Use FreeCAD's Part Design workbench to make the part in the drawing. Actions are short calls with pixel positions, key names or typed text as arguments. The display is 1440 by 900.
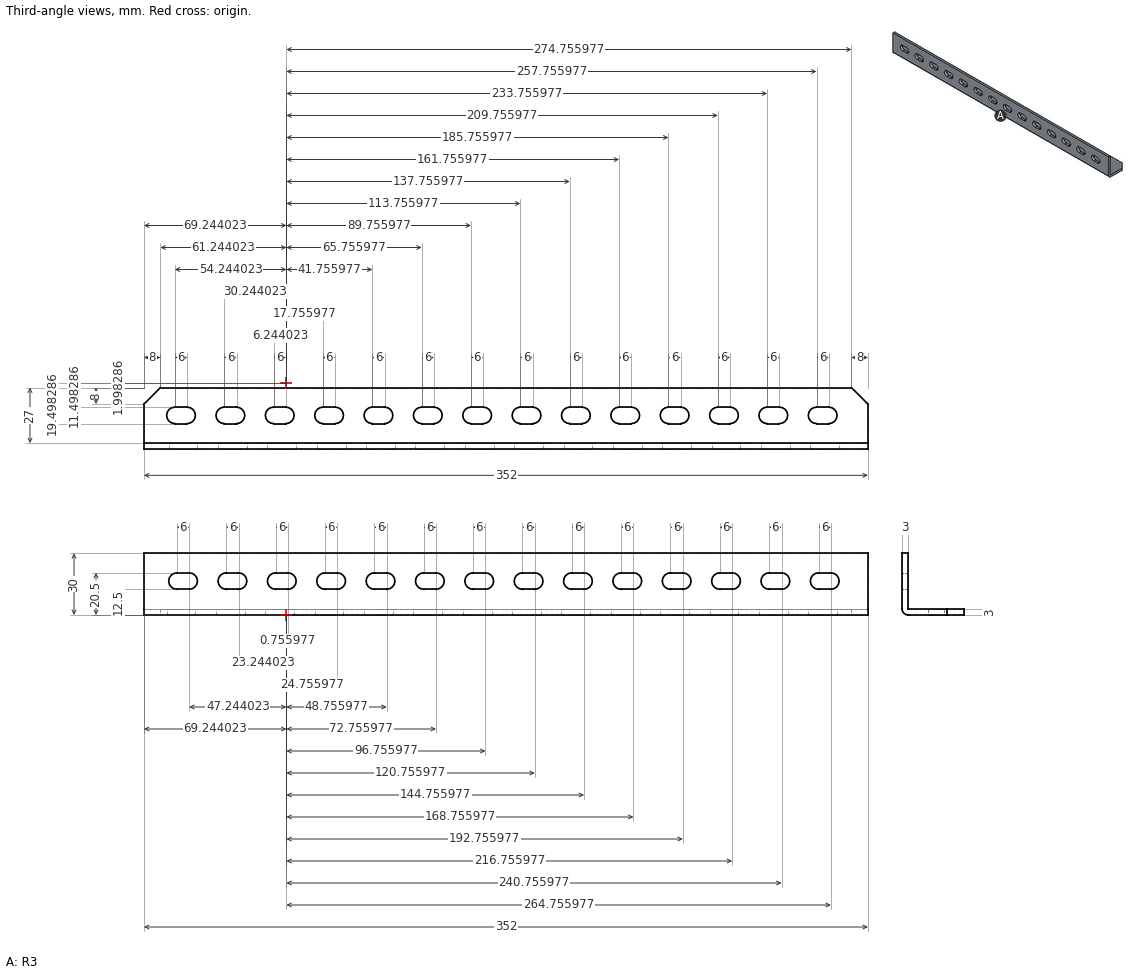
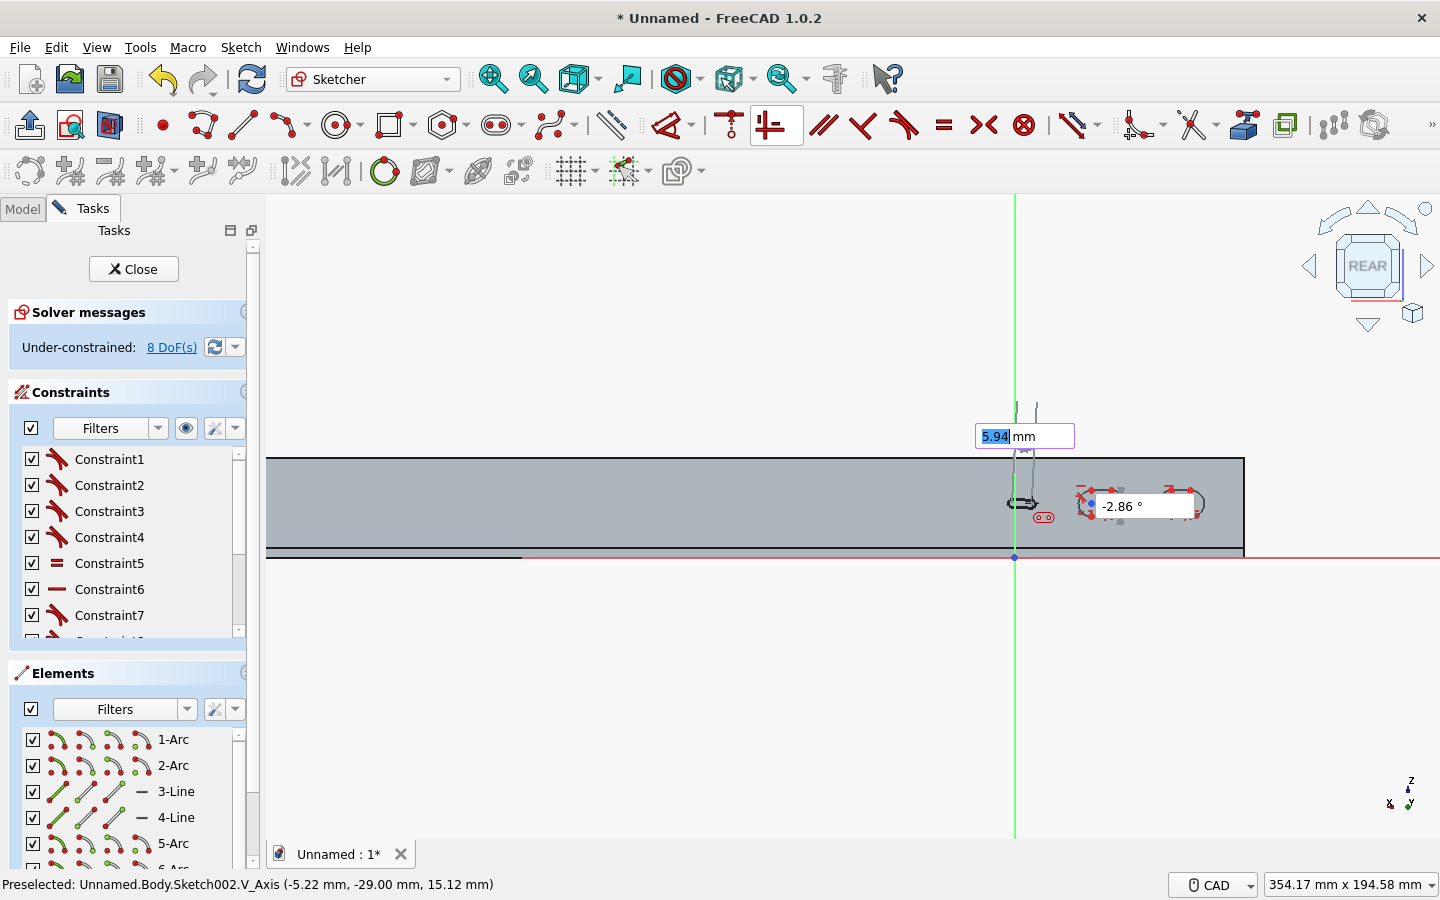
click(1032, 503)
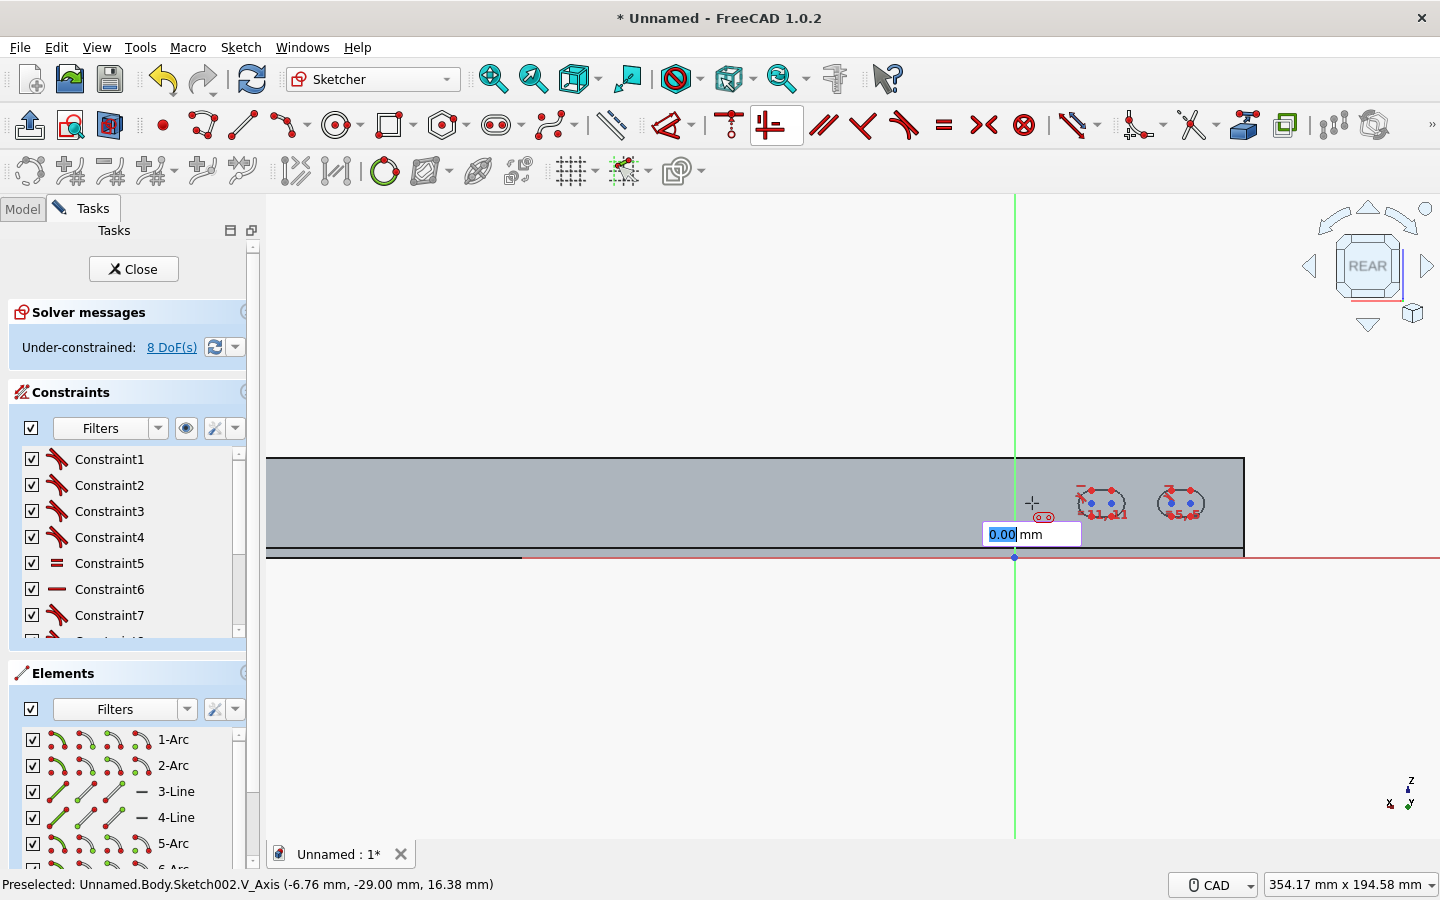
scroll(1025, 516, up, 3)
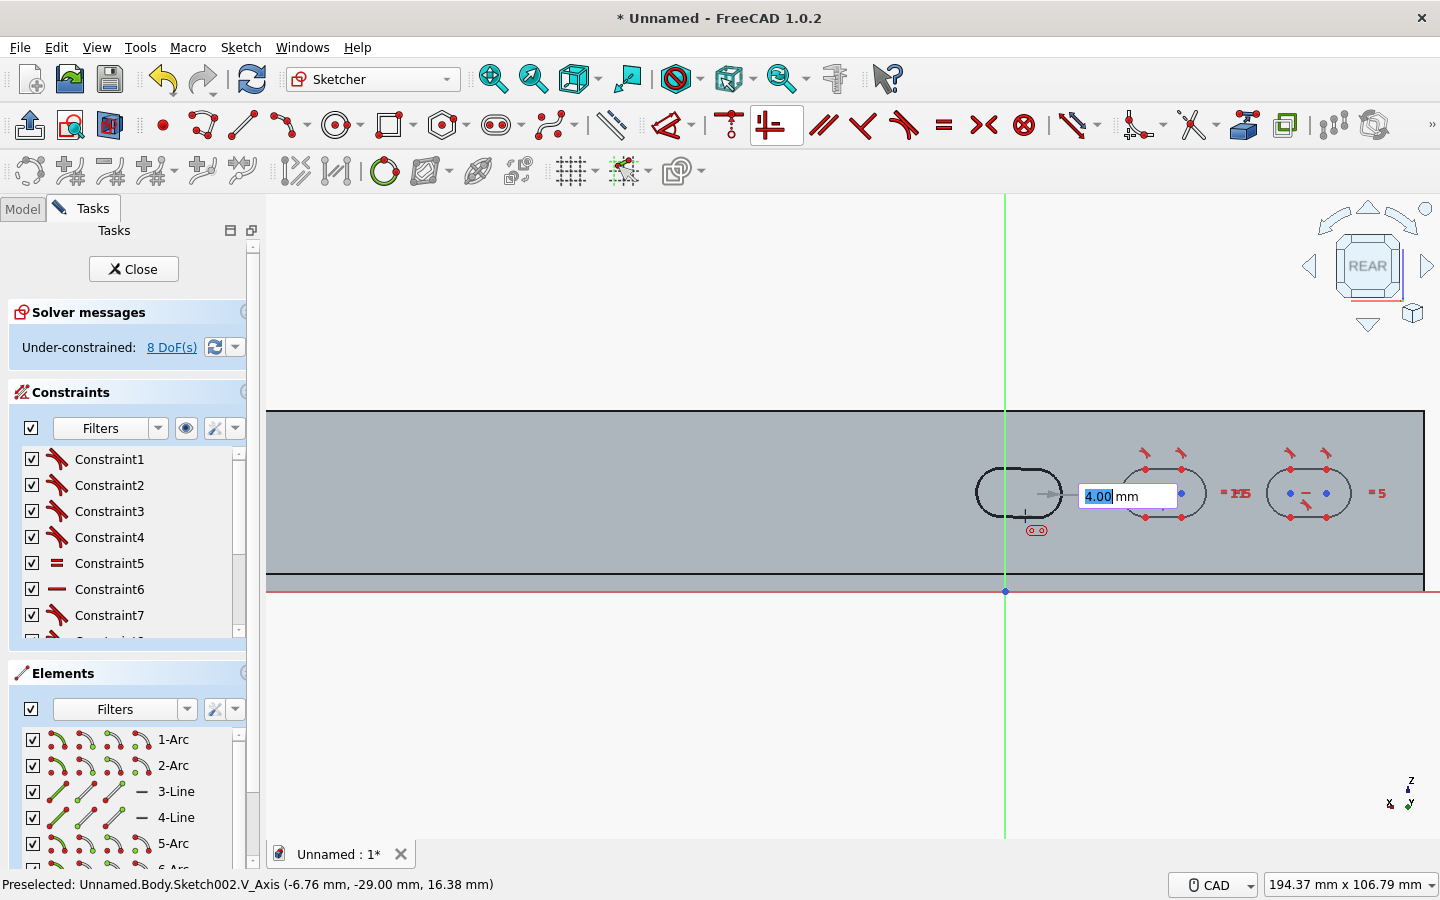
click(1024, 516)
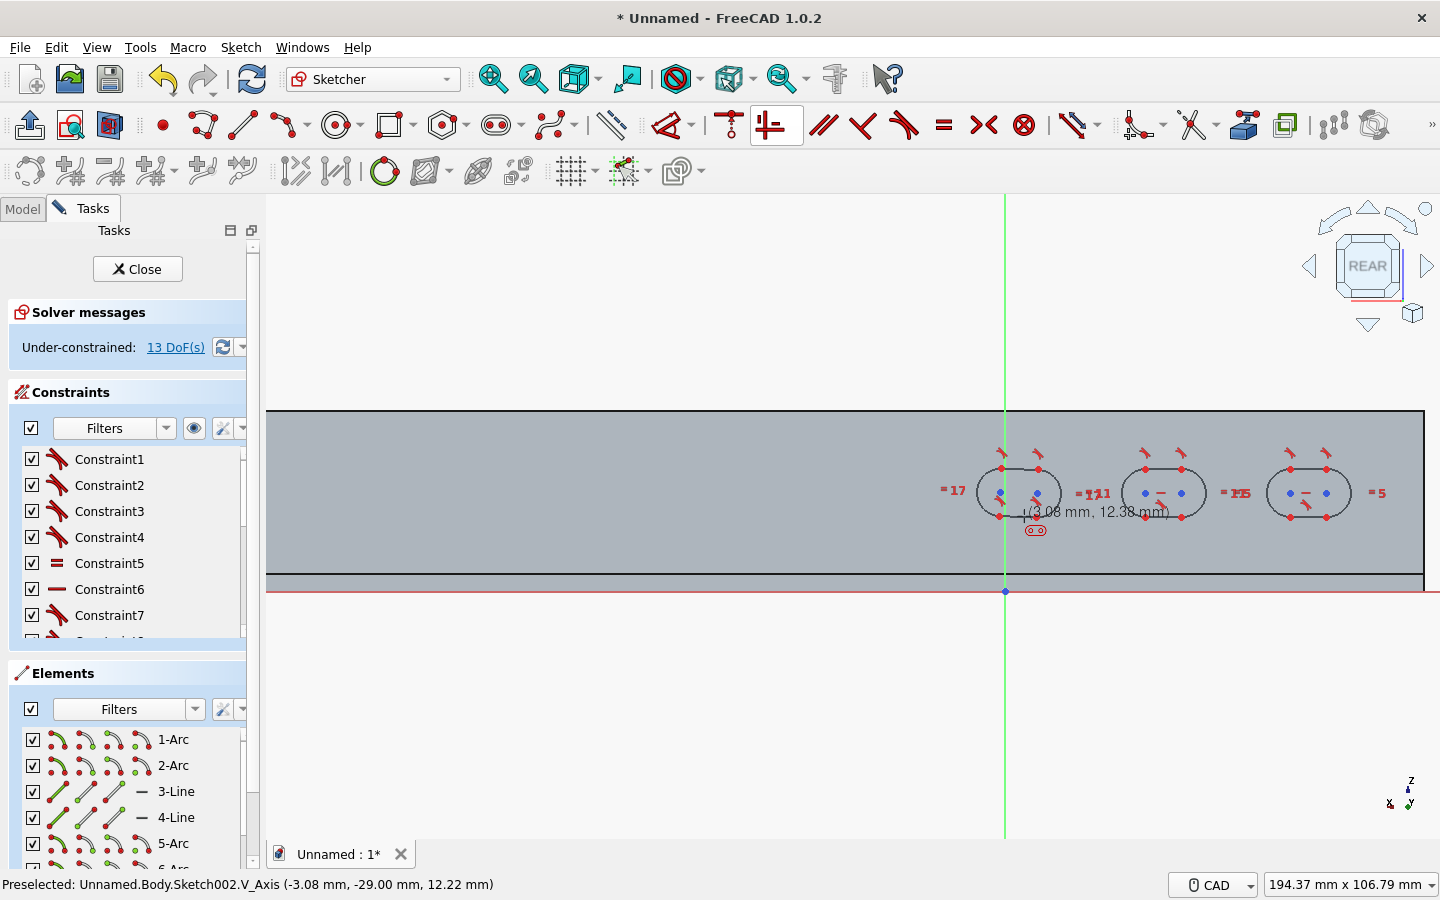
click(856, 492)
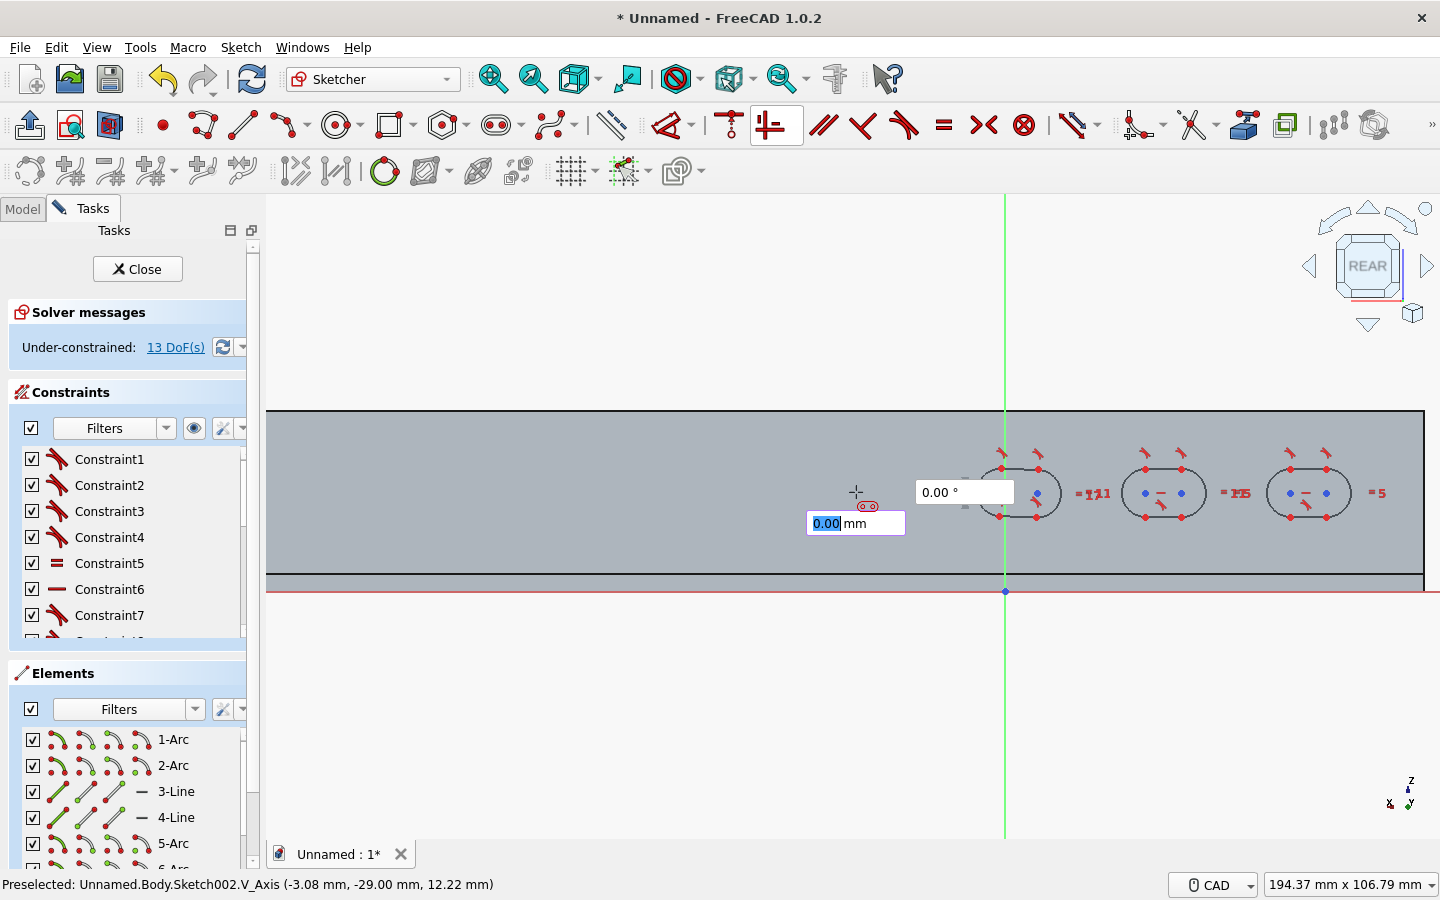
click(892, 492)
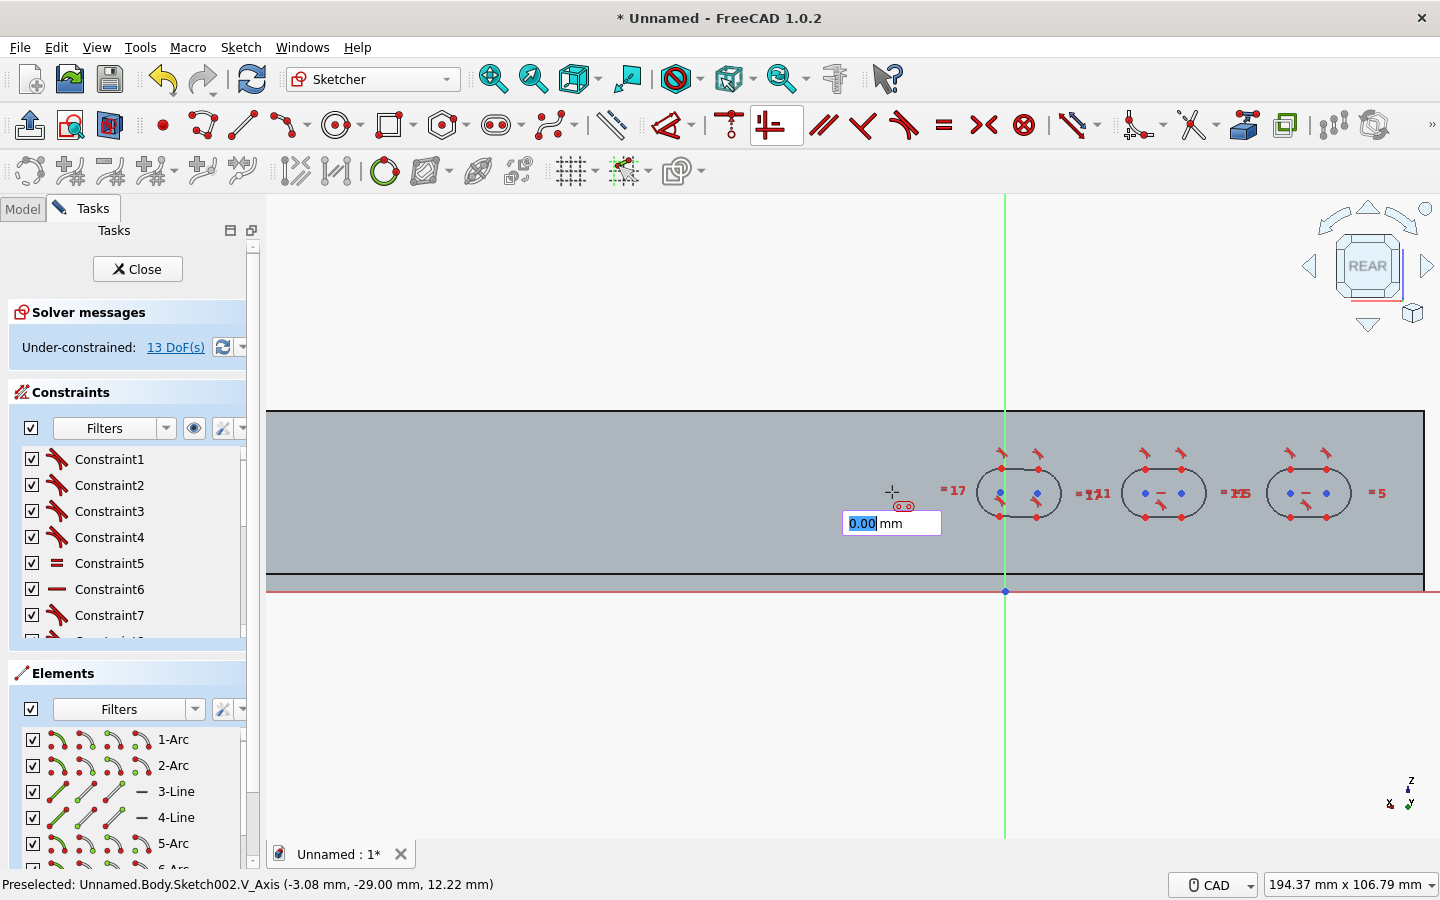
click(874, 516)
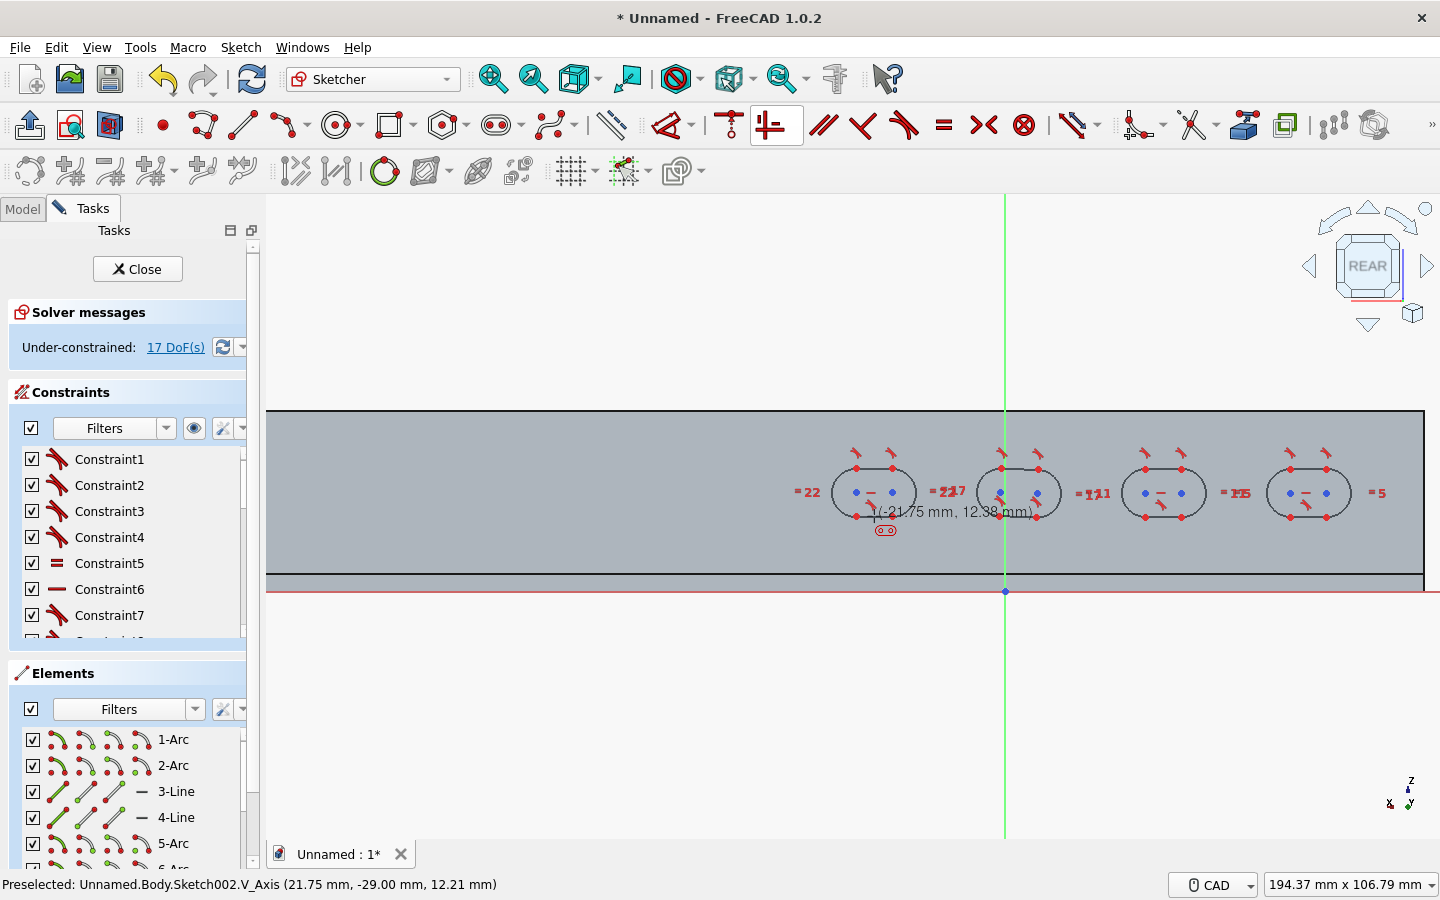
click(711, 492)